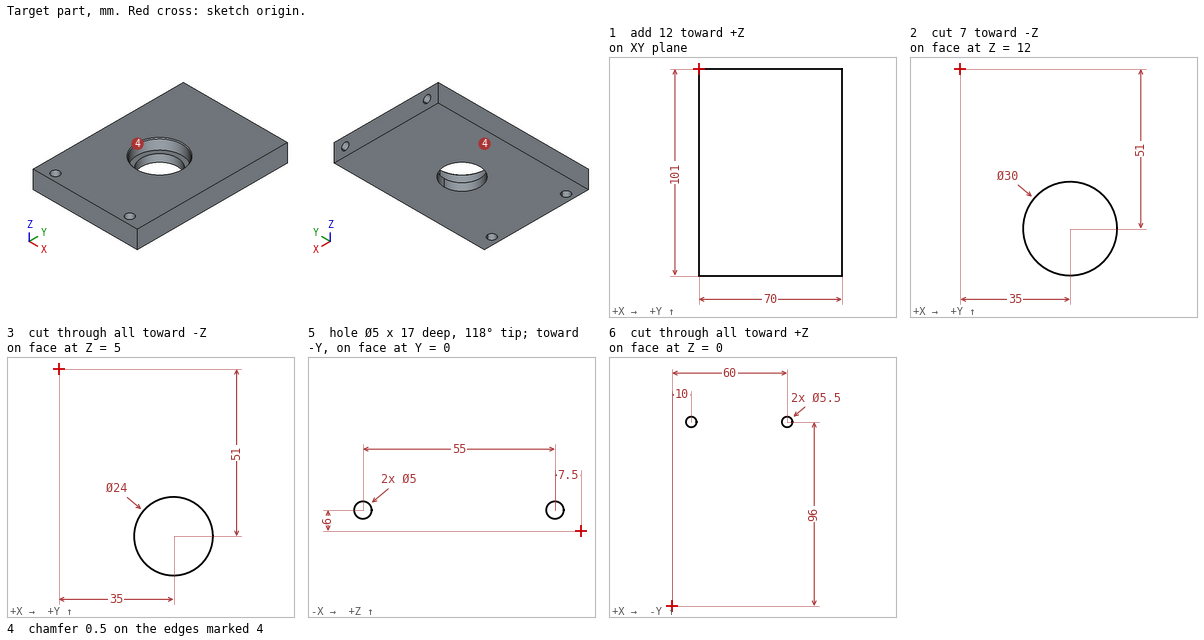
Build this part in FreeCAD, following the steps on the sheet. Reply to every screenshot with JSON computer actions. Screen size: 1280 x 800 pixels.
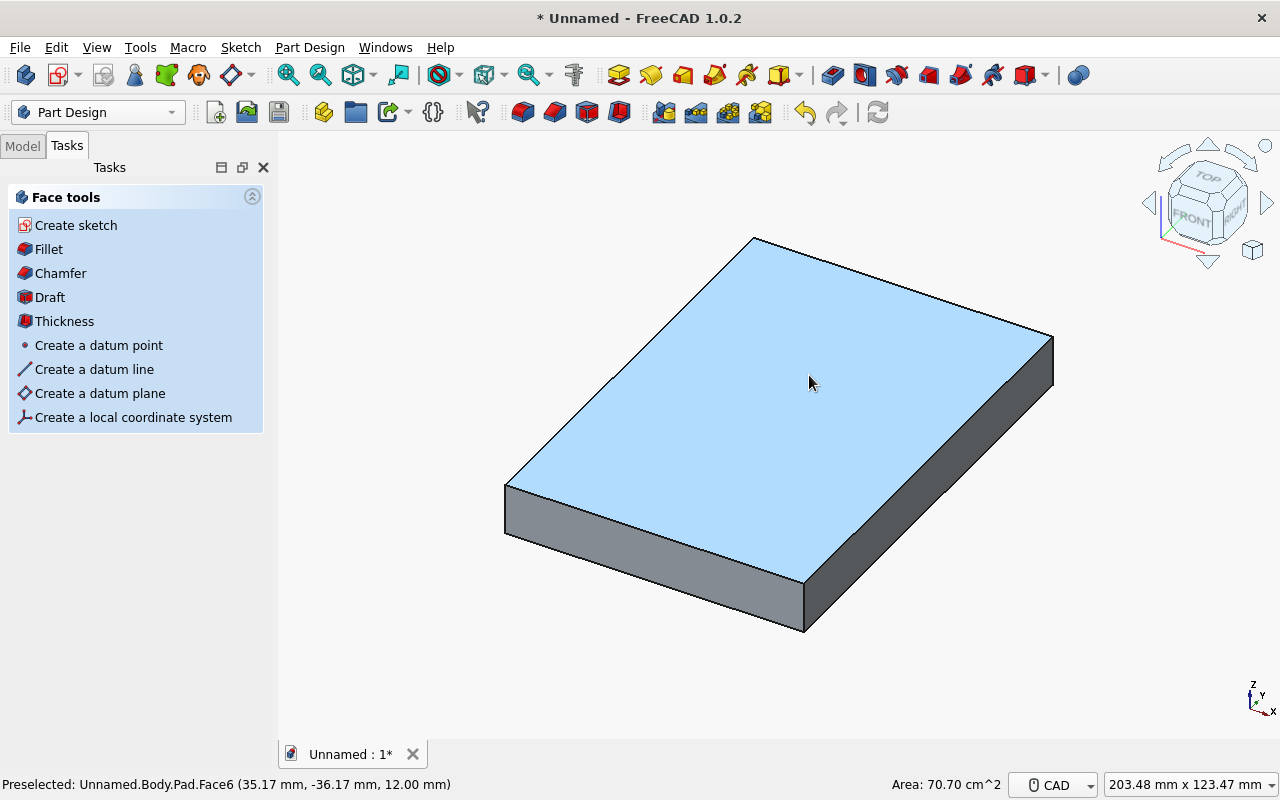
{"action": "left_click", "coordinate": [58, 76]}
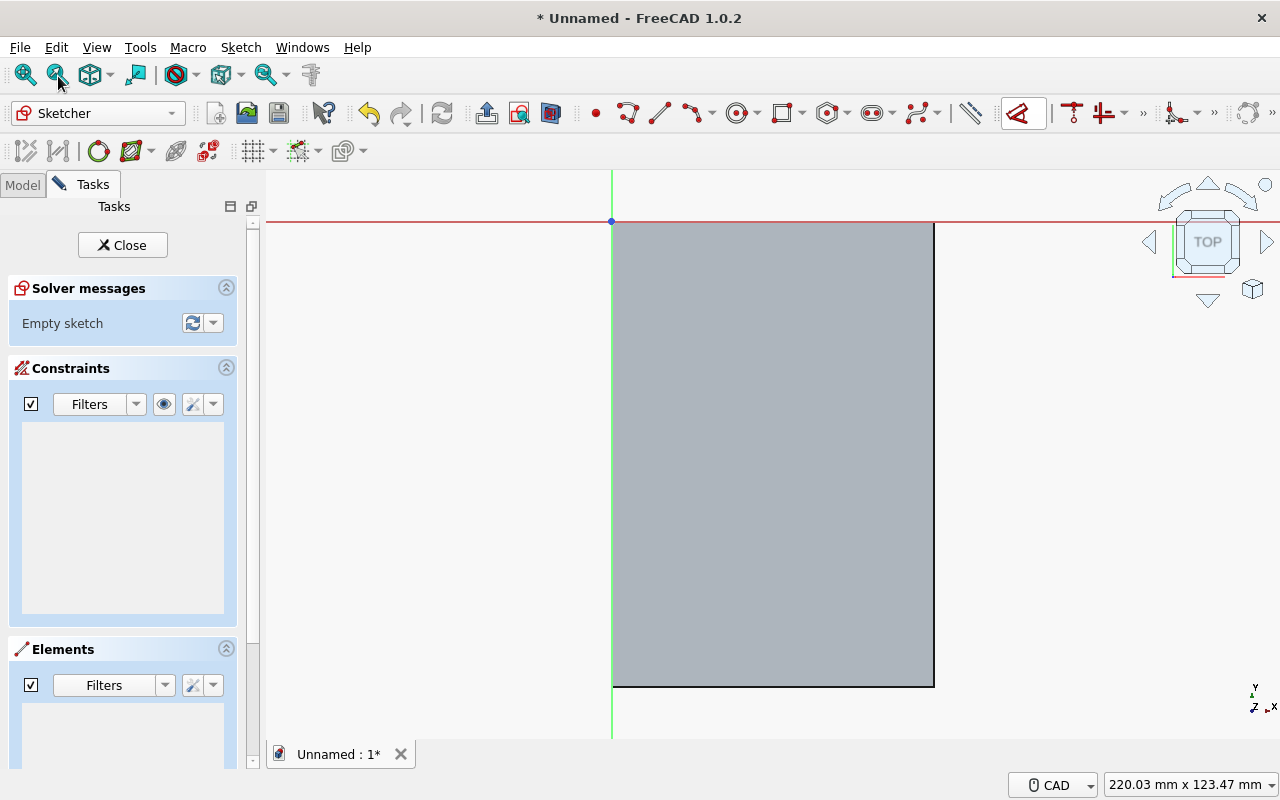
{"action": "scroll", "coordinate": [828, 198], "scroll_direction": "up", "scroll_amount": 1}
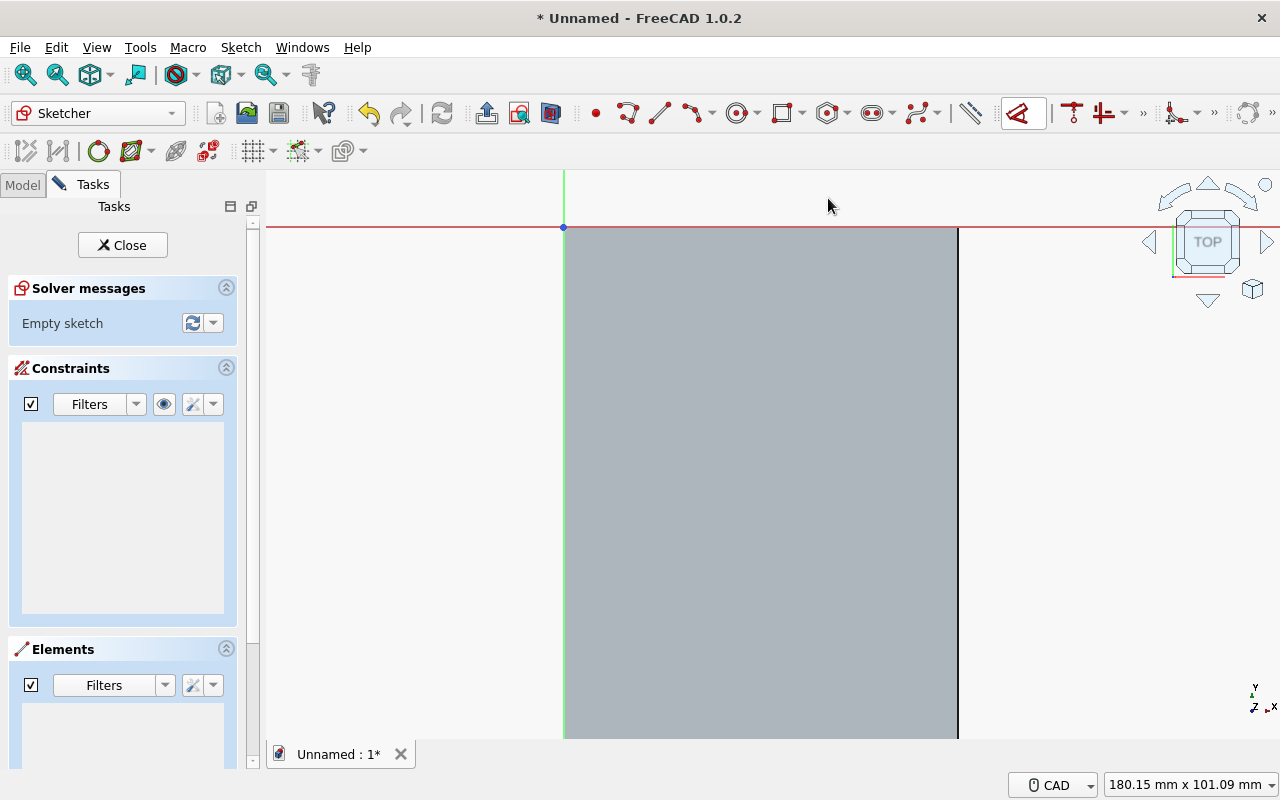
{"action": "left_click", "coordinate": [738, 114]}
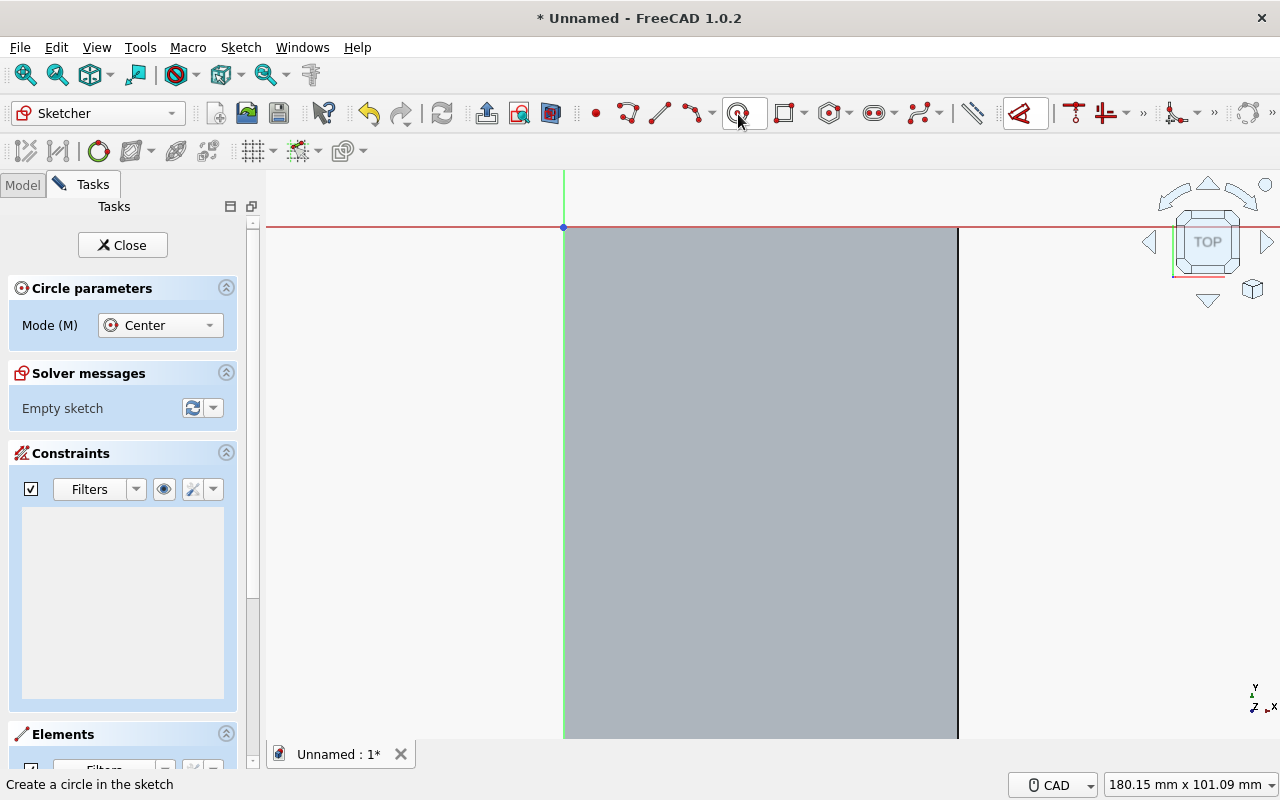
{"action": "left_click", "coordinate": [761, 514]}
{"action": "left_click", "coordinate": [820, 454]}
{"action": "key", "text": "Escape"}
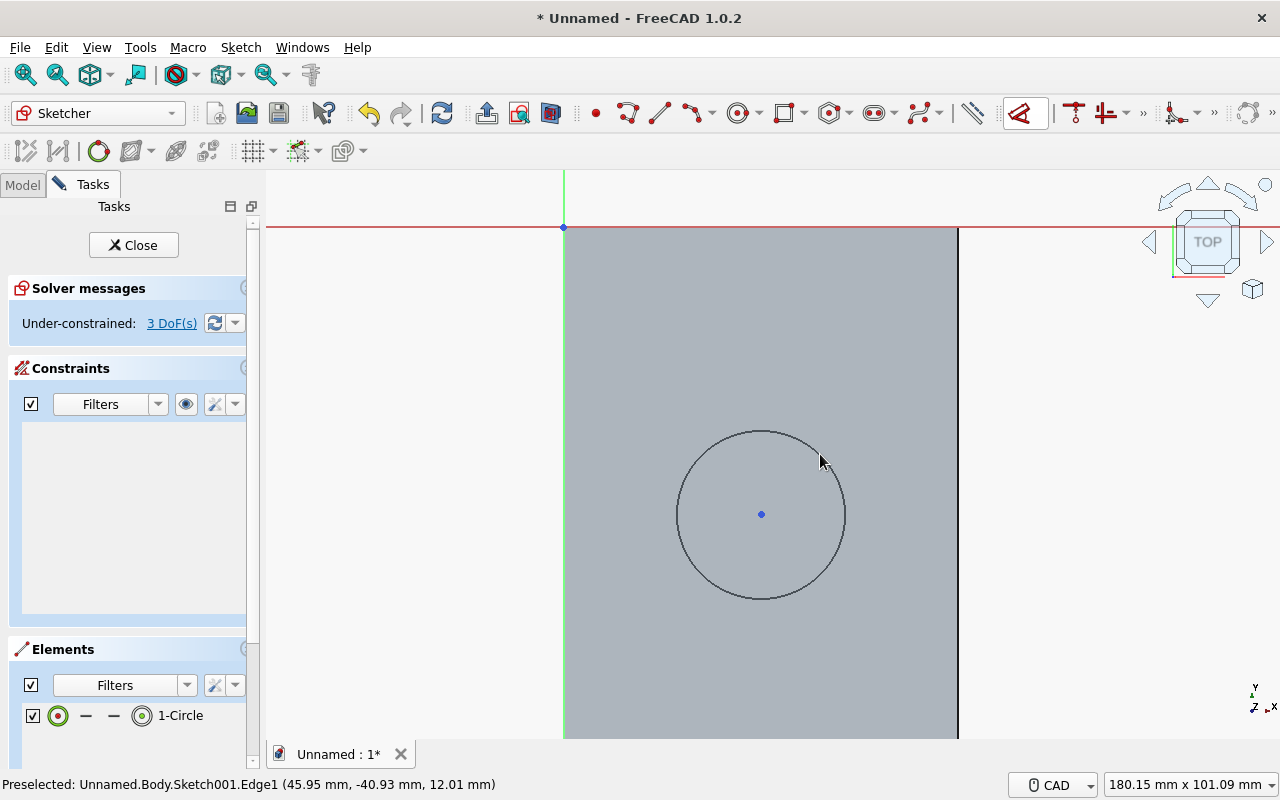
{"action": "left_click", "coordinate": [820, 455]}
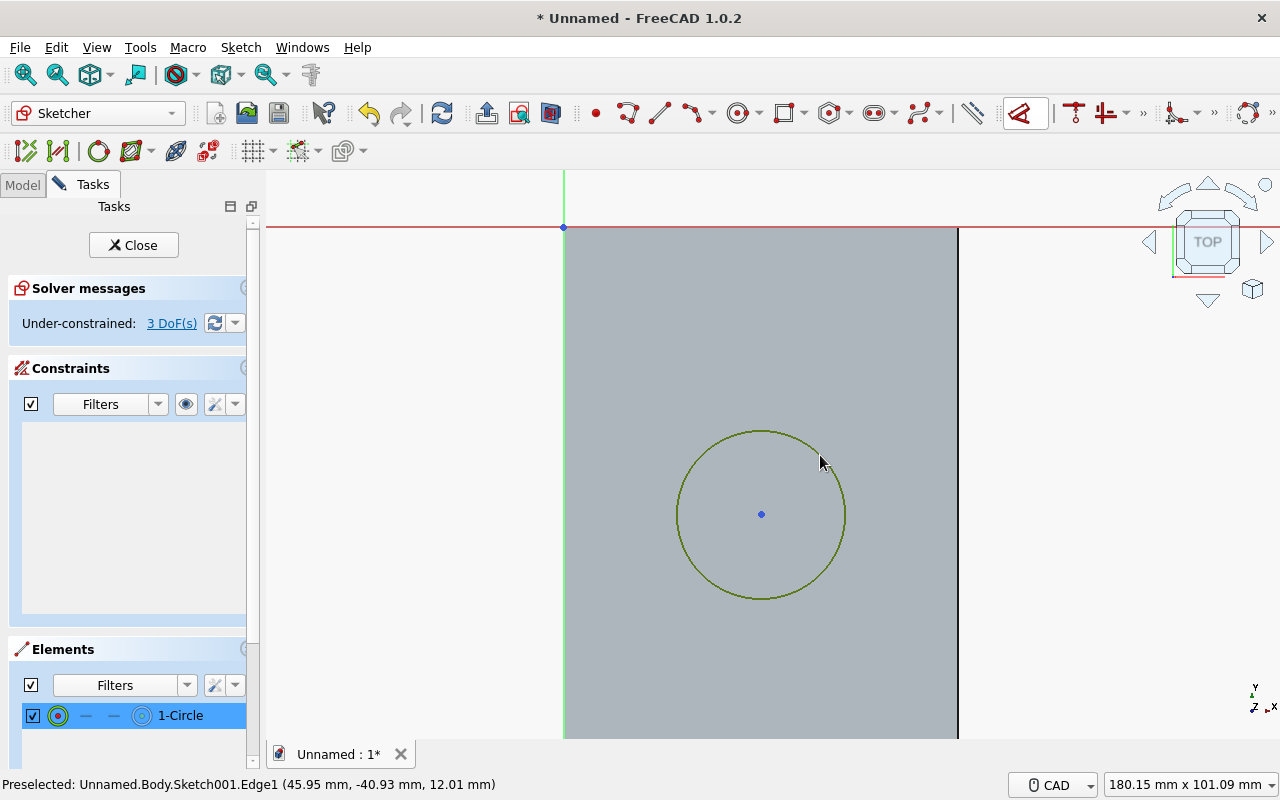
{"action": "key", "text": "k o"}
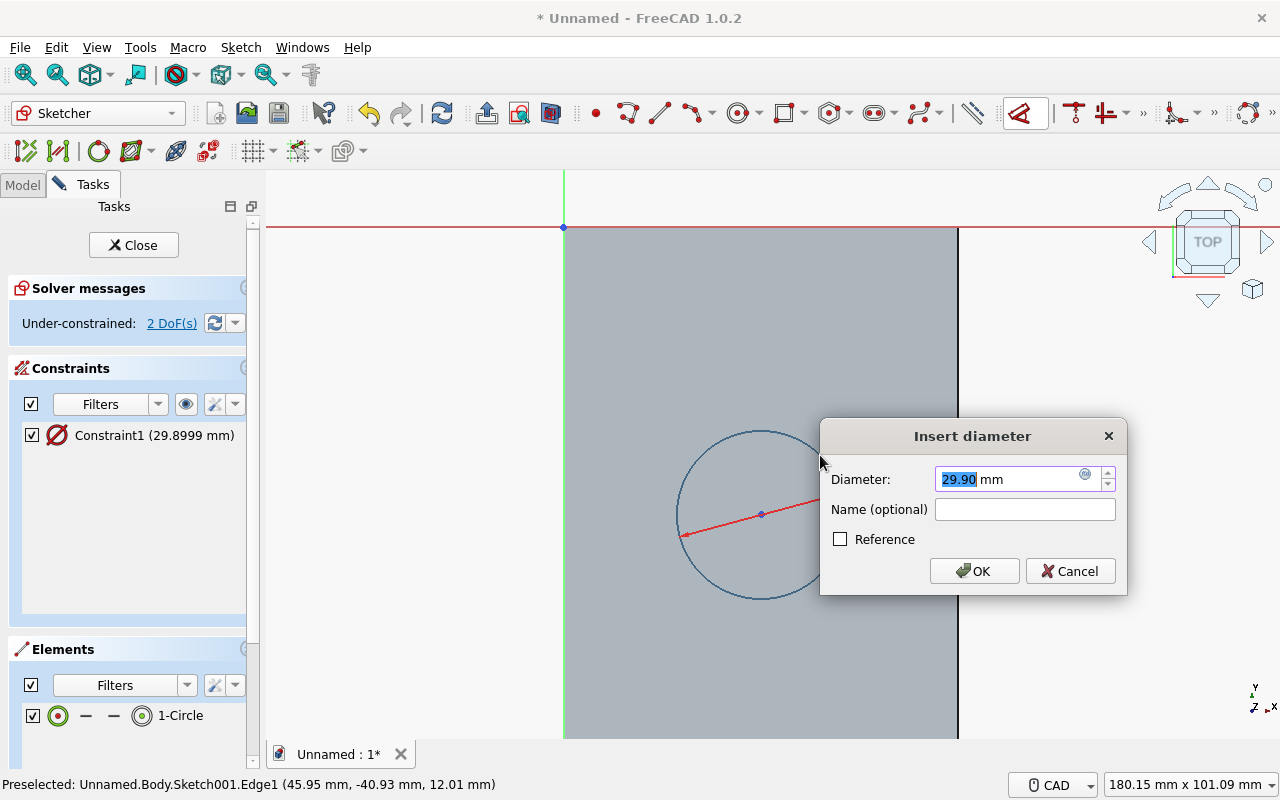
{"action": "type", "text": "30"}
{"action": "key", "text": "Return"}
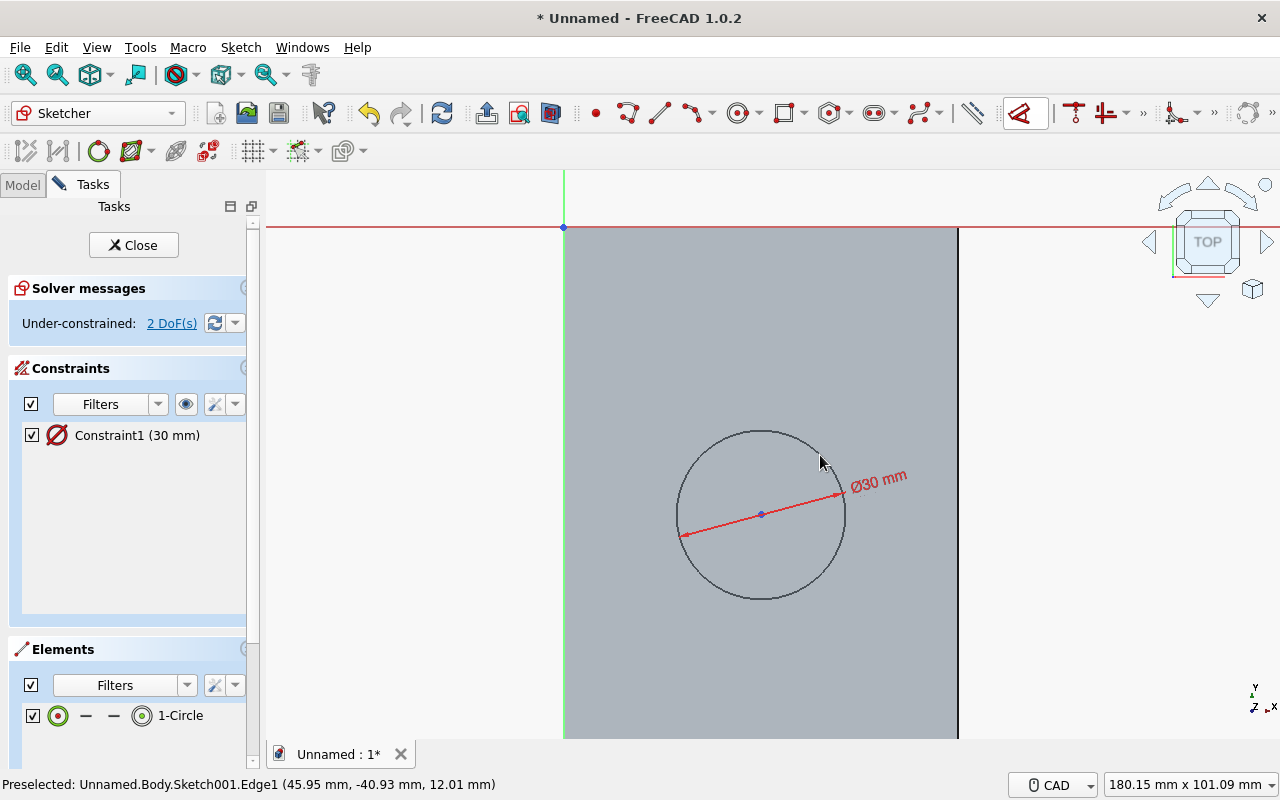
{"action": "left_click", "coordinate": [761, 515]}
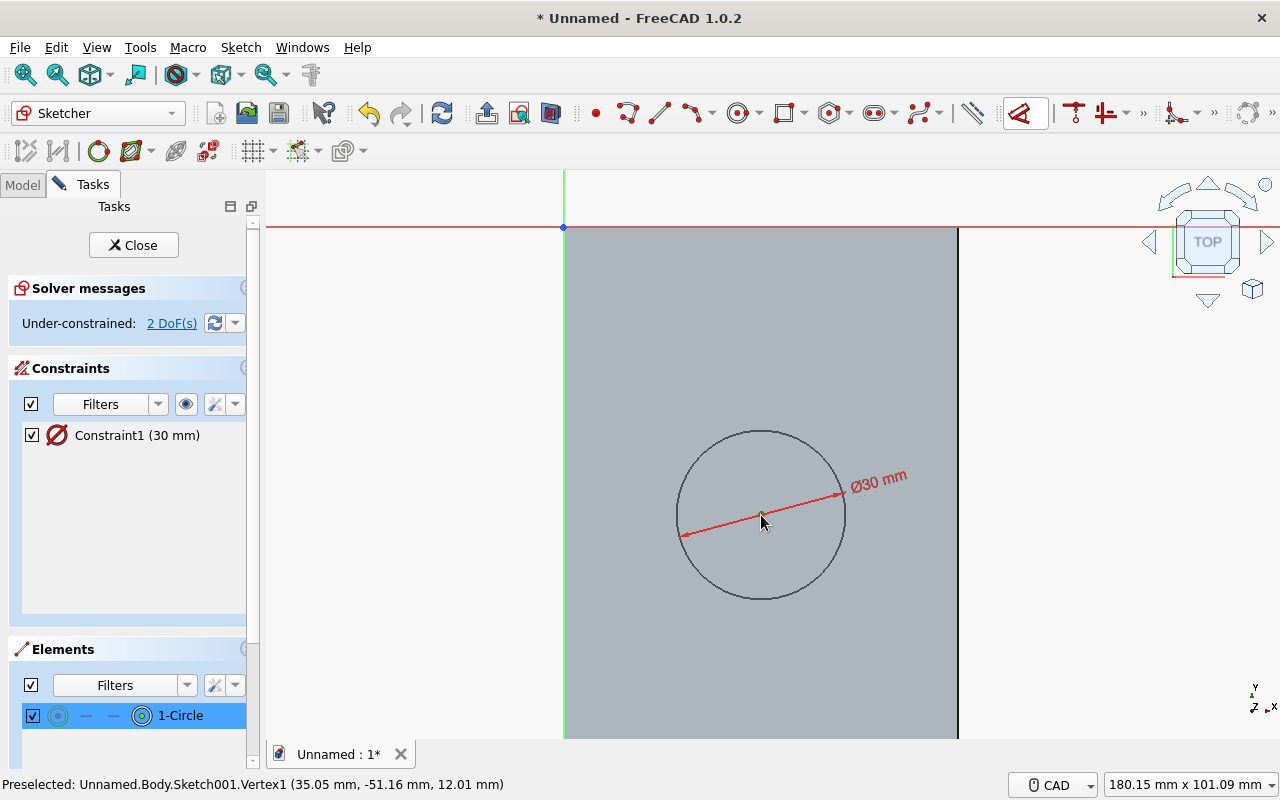
{"action": "key", "text": "l"}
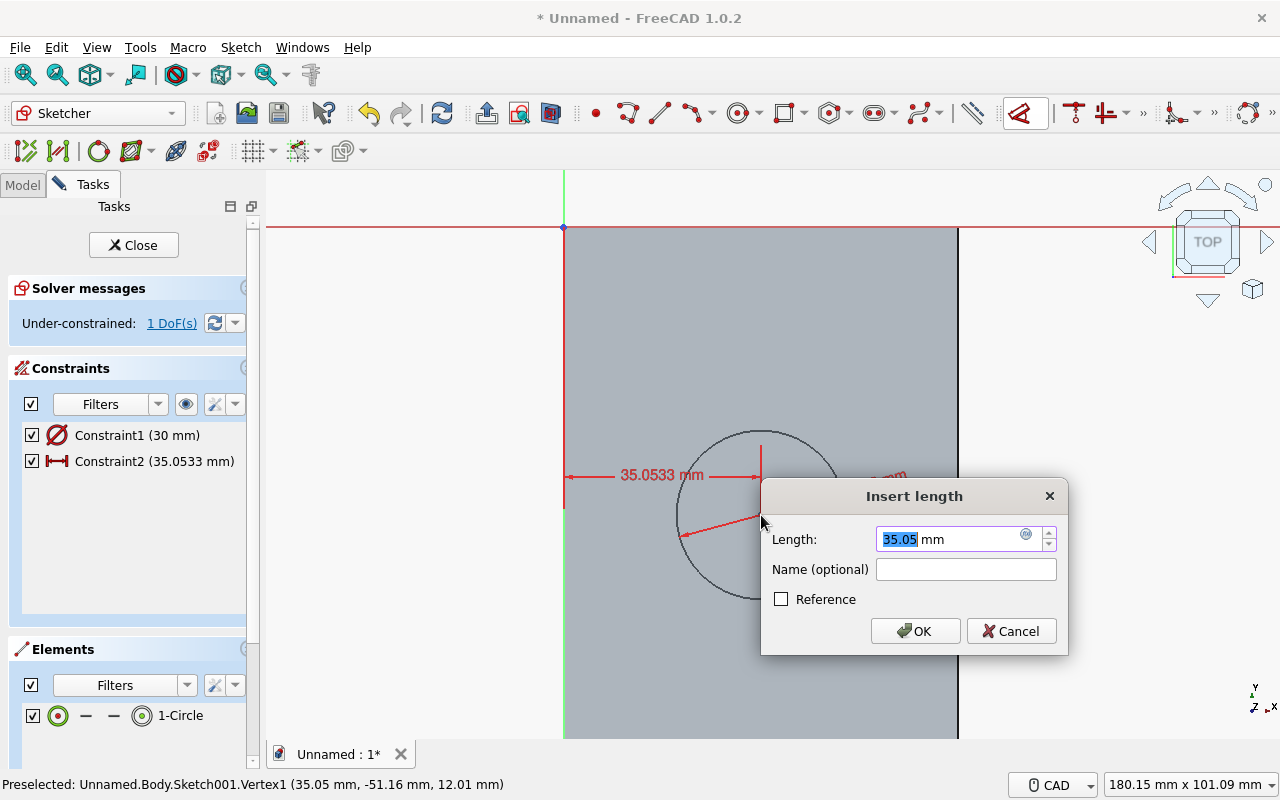
{"action": "type", "text": "35"}
{"action": "key", "text": "Return"}